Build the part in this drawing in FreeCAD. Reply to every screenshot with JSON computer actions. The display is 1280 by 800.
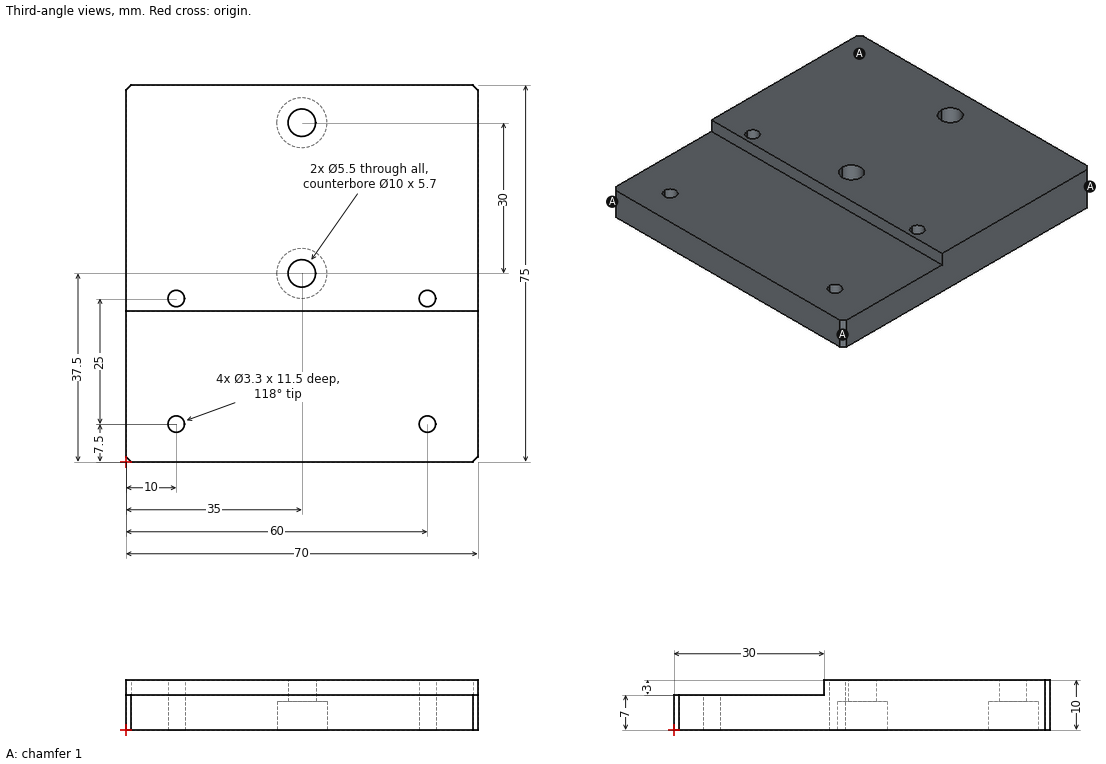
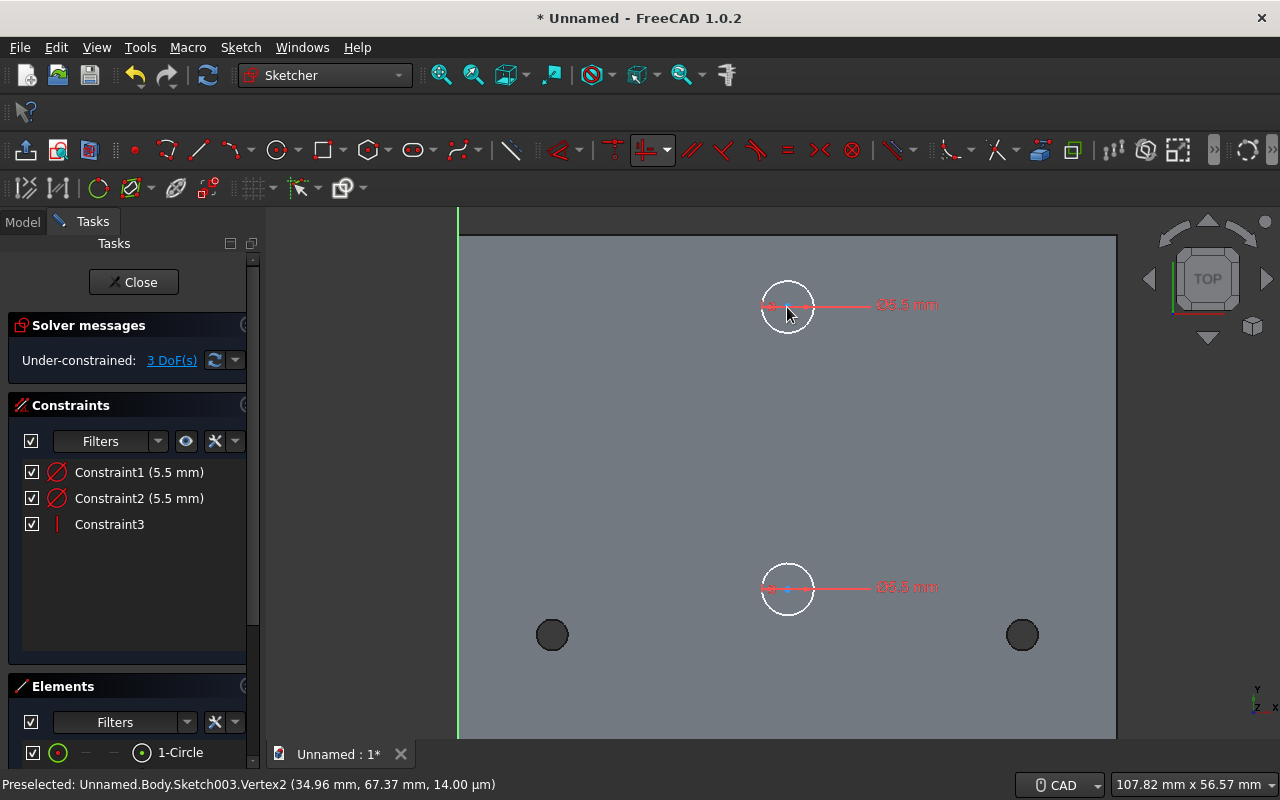
{"action": "left_click", "coordinate": [558, 150]}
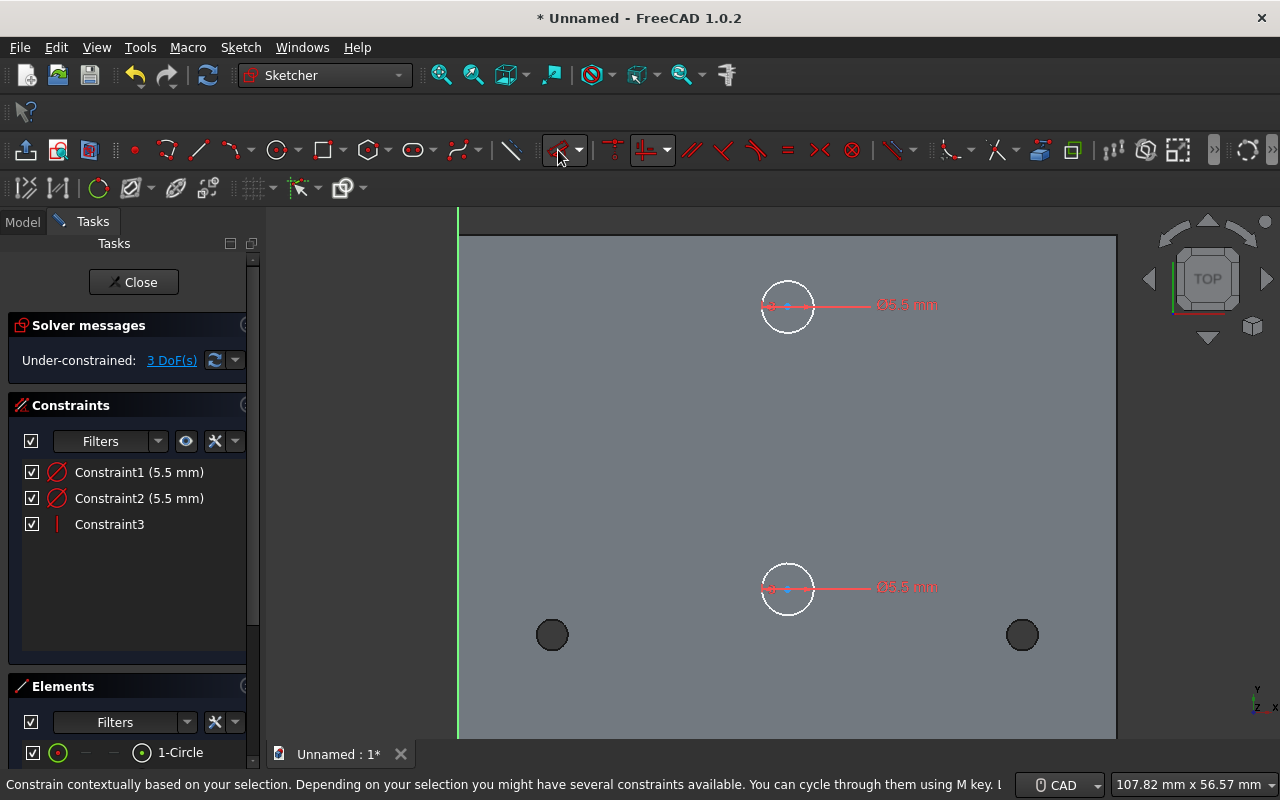
{"action": "left_click", "coordinate": [788, 589]}
{"action": "left_click", "coordinate": [623, 555]}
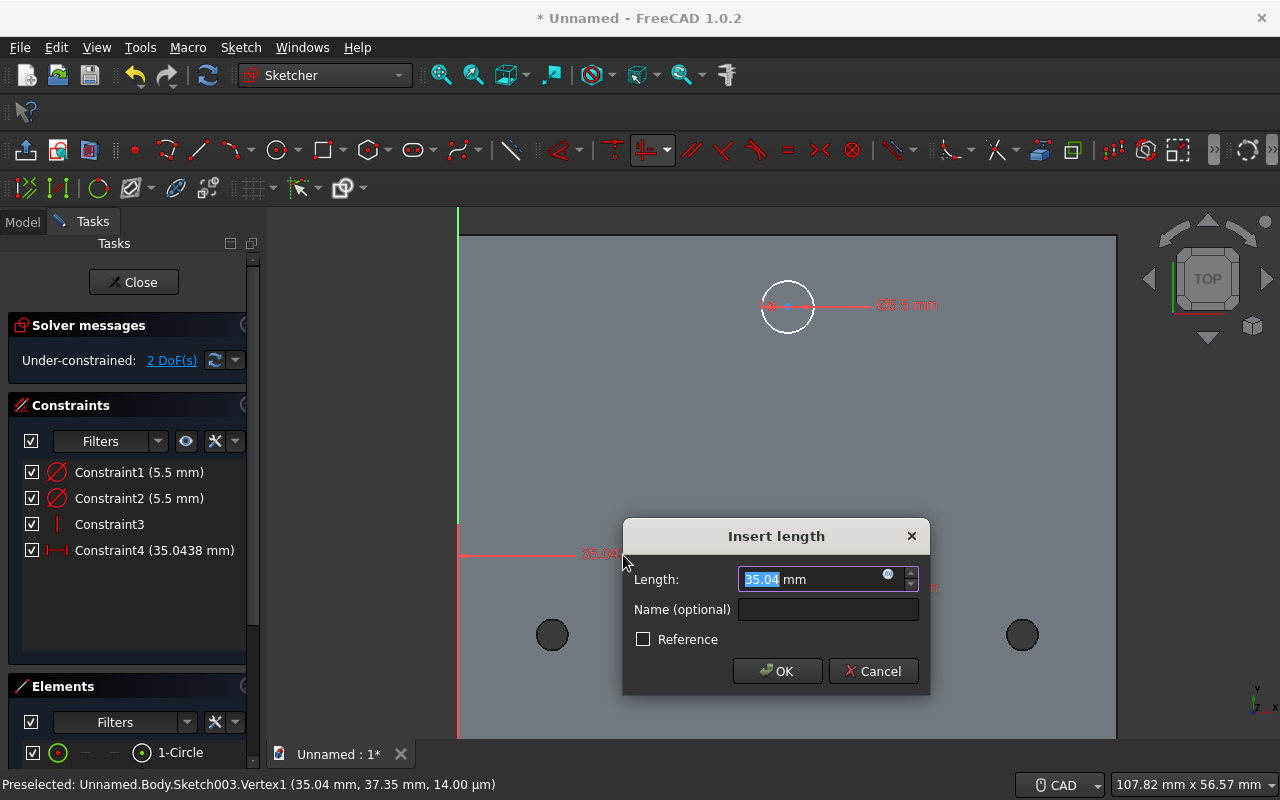
{"action": "type", "text": "35"}
{"action": "key", "text": "Return"}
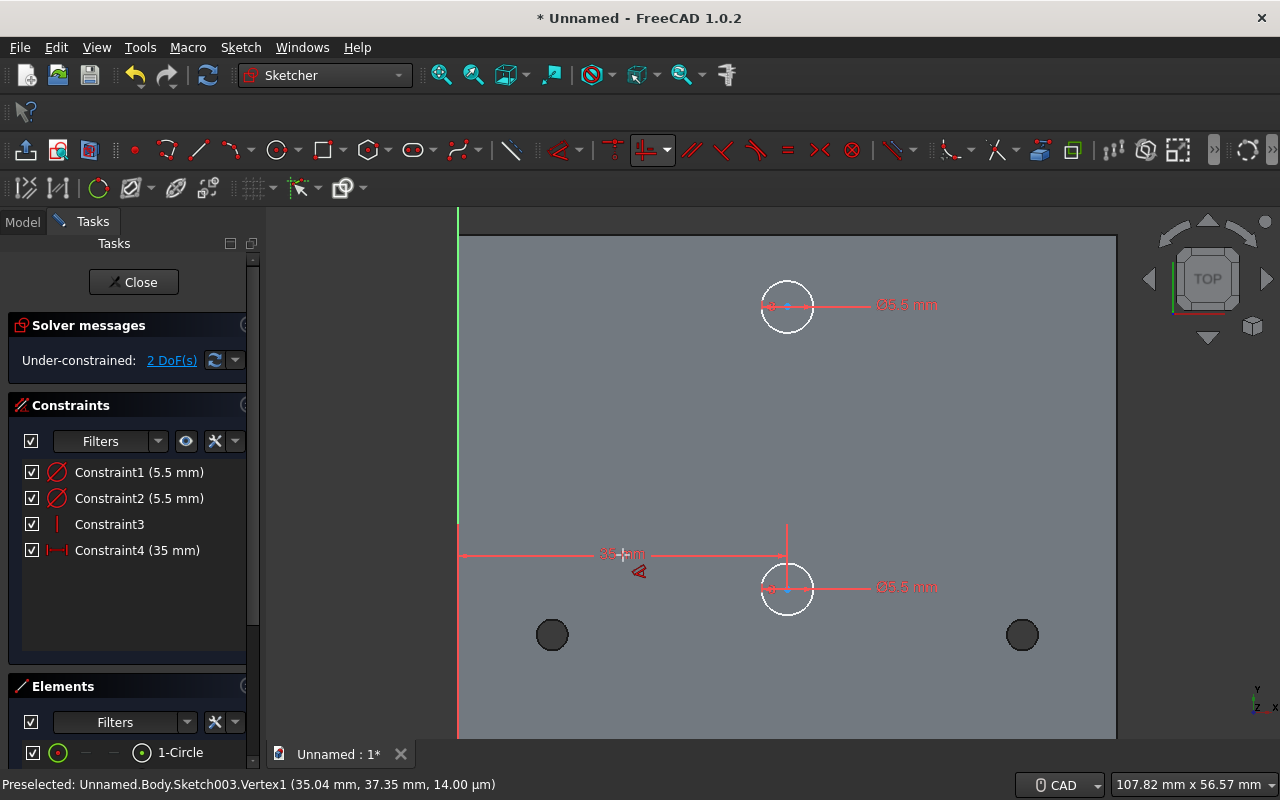
{"action": "left_click", "coordinate": [787, 589]}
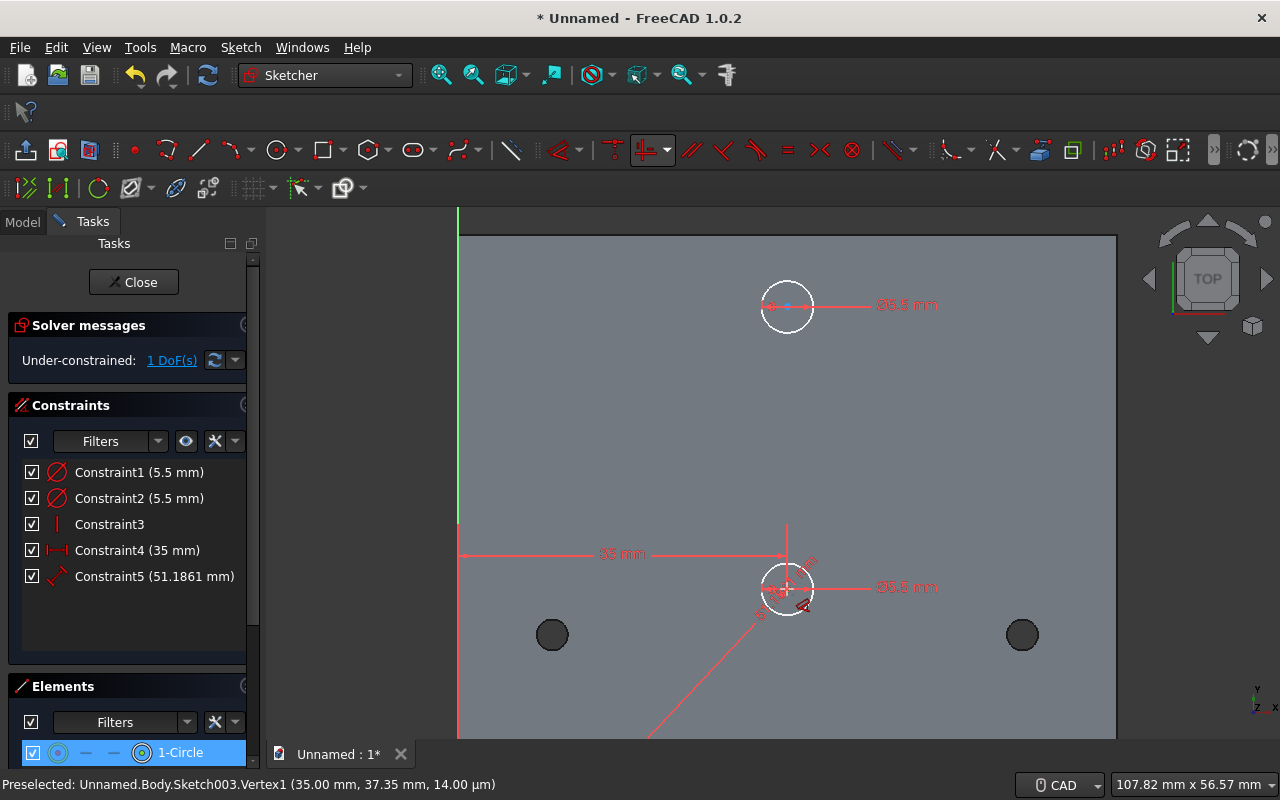
{"action": "left_click", "coordinate": [787, 307]}
{"action": "left_click", "coordinate": [821, 448]}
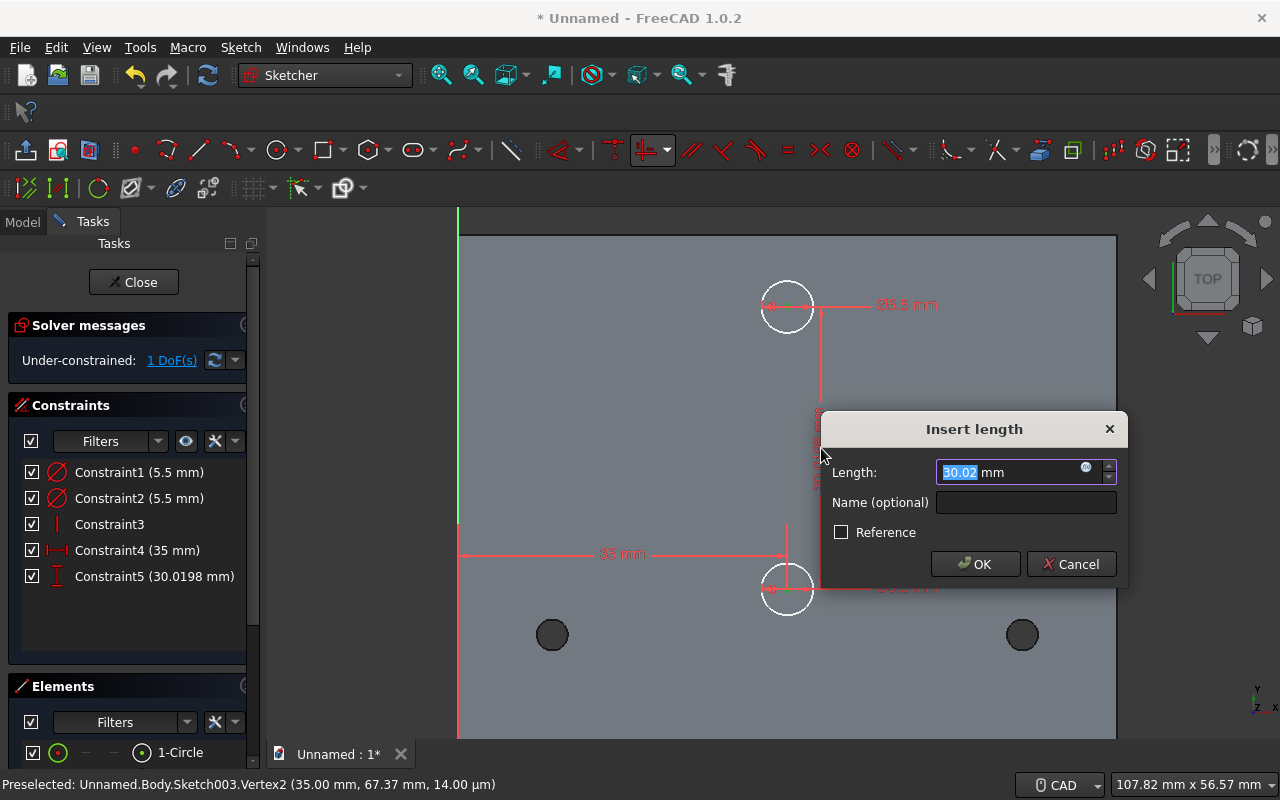
{"action": "type", "text": "30"}
{"action": "key", "text": "Return"}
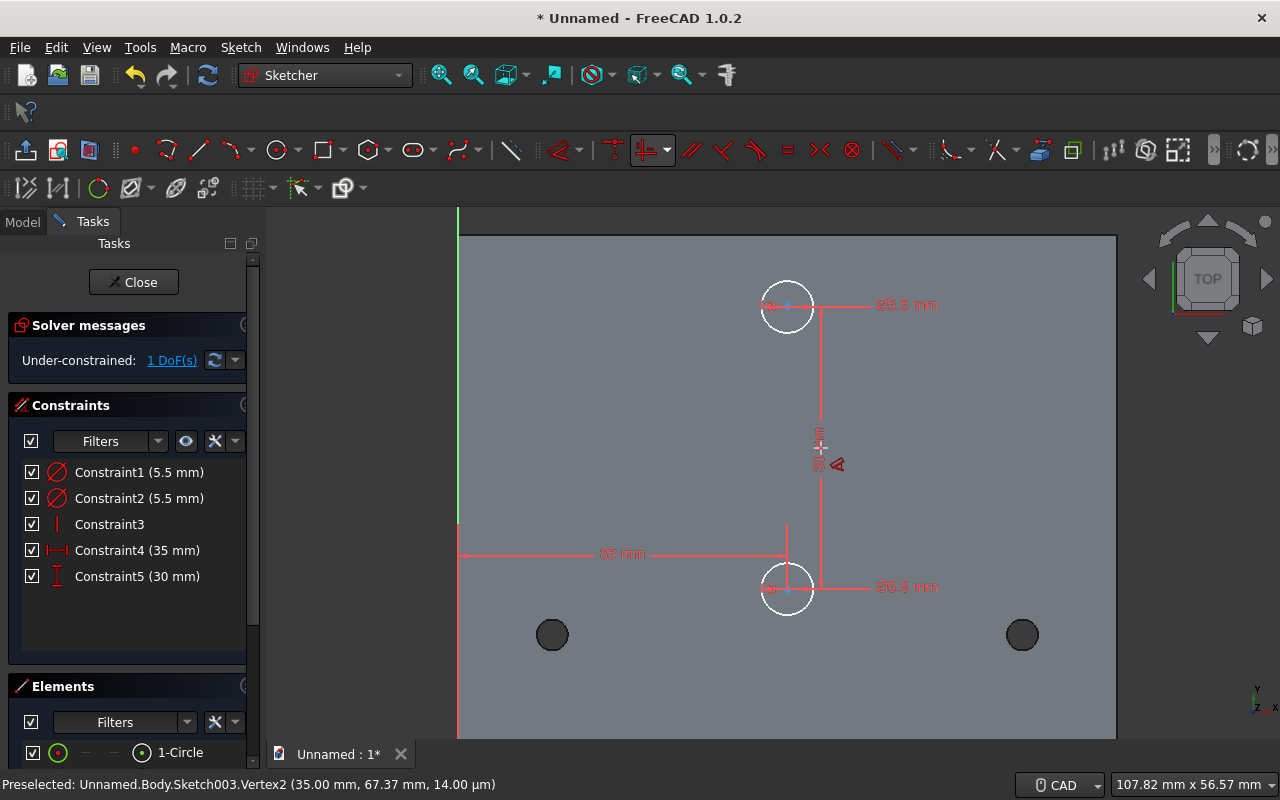
{"action": "left_click", "coordinate": [787, 589]}
{"action": "left_click", "coordinate": [424, 650]}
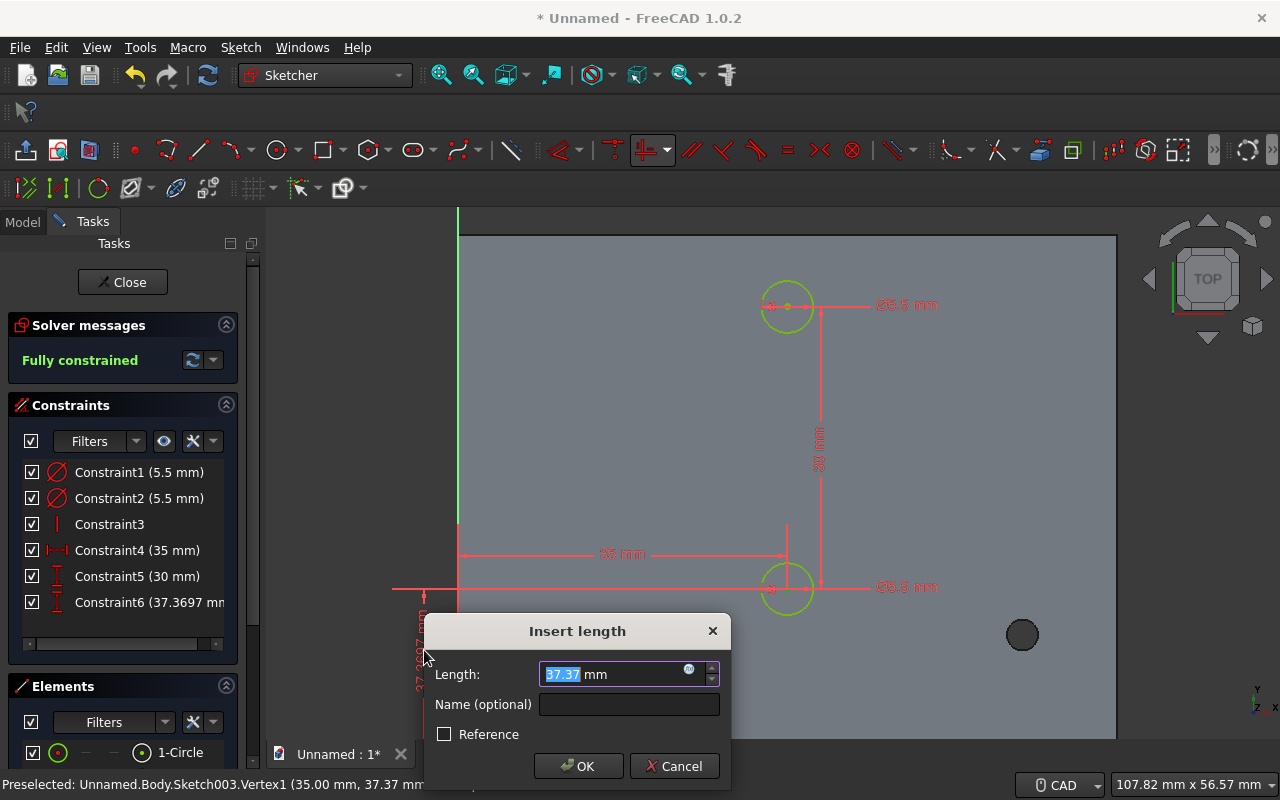
{"action": "type", "text": "37.5"}
{"action": "key", "text": "Return"}
{"action": "key", "text": "Escape"}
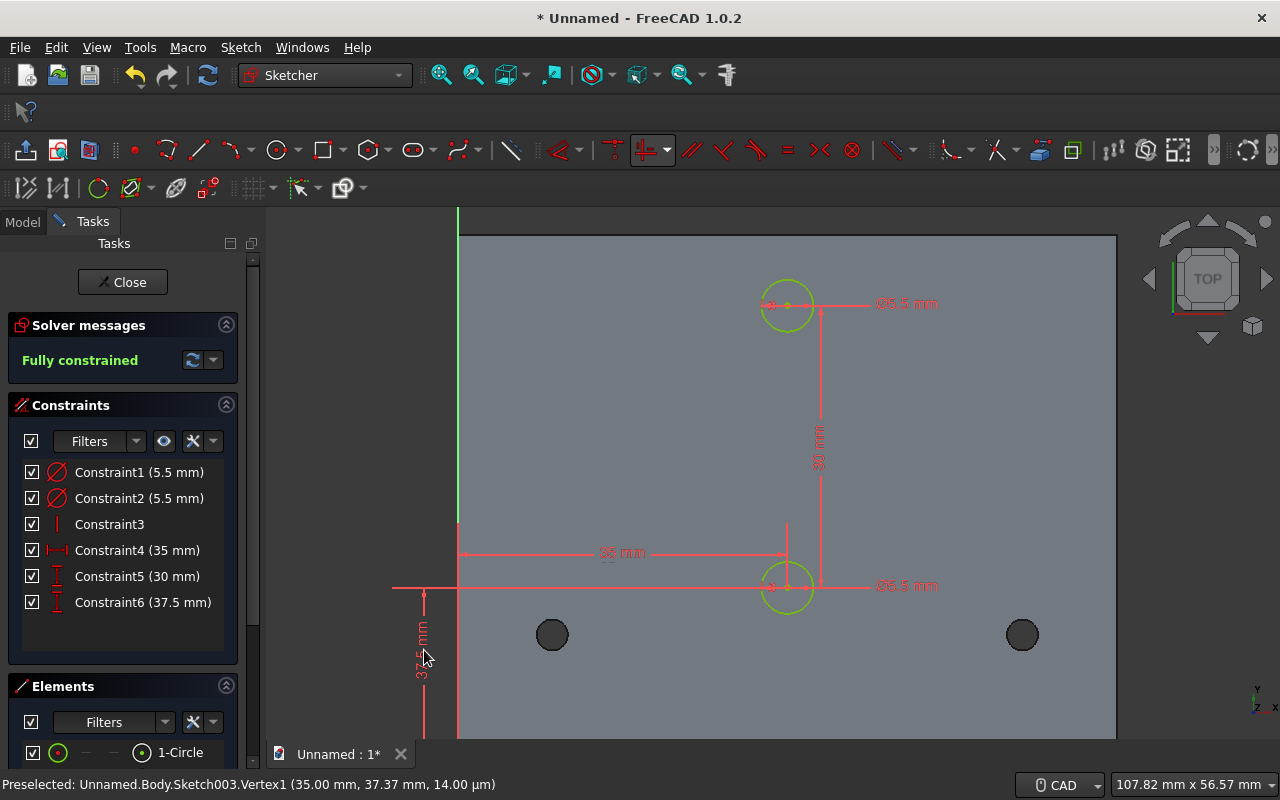
{"action": "left_click", "coordinate": [123, 282]}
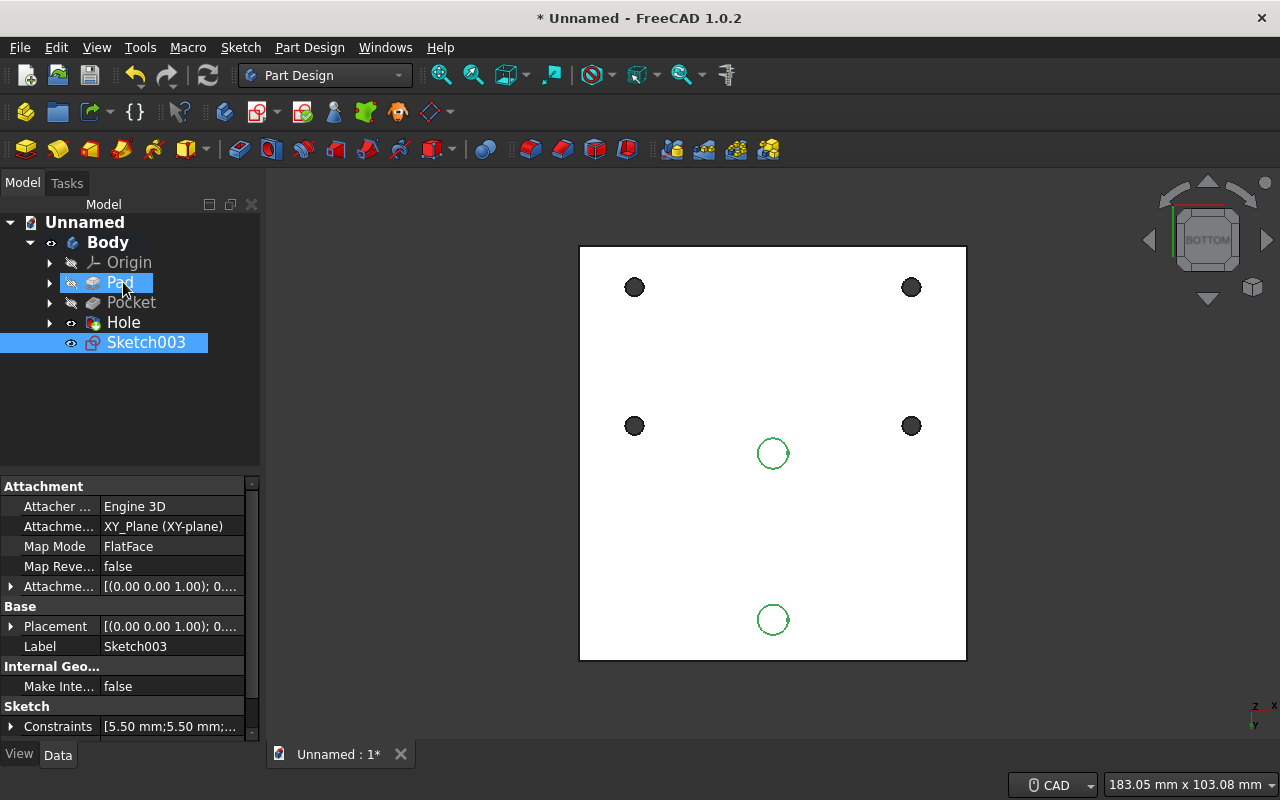
{"action": "left_click", "coordinate": [272, 150]}